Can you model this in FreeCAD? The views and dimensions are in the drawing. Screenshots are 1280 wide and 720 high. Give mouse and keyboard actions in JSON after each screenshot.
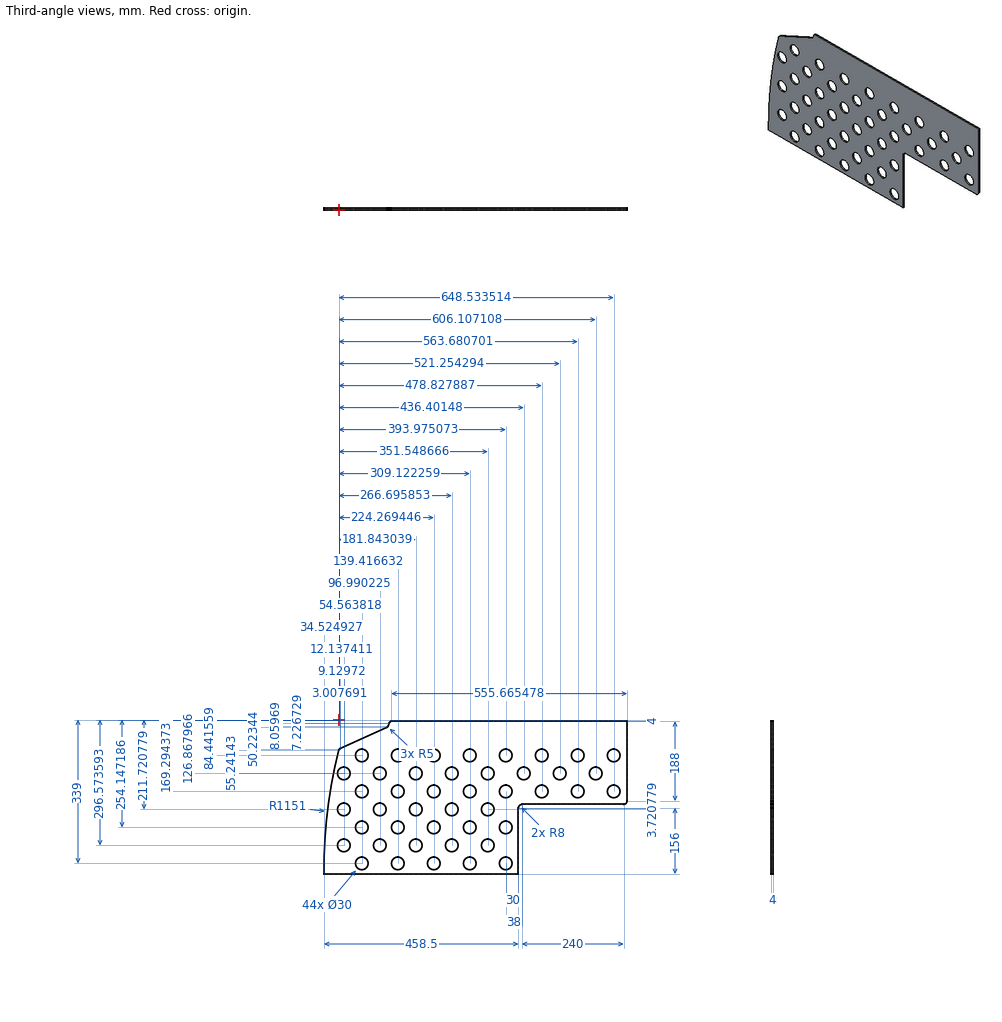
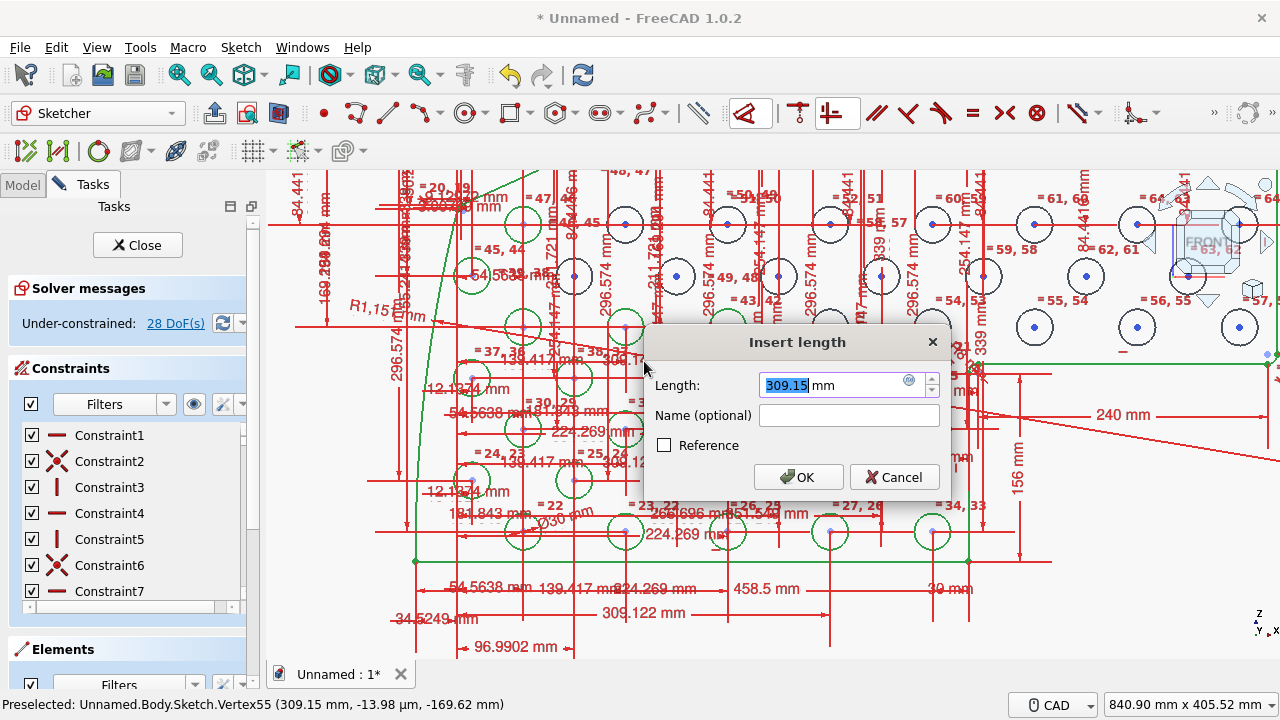
{"action": "type", "text": "309.122259"}
{"action": "key", "text": "Return"}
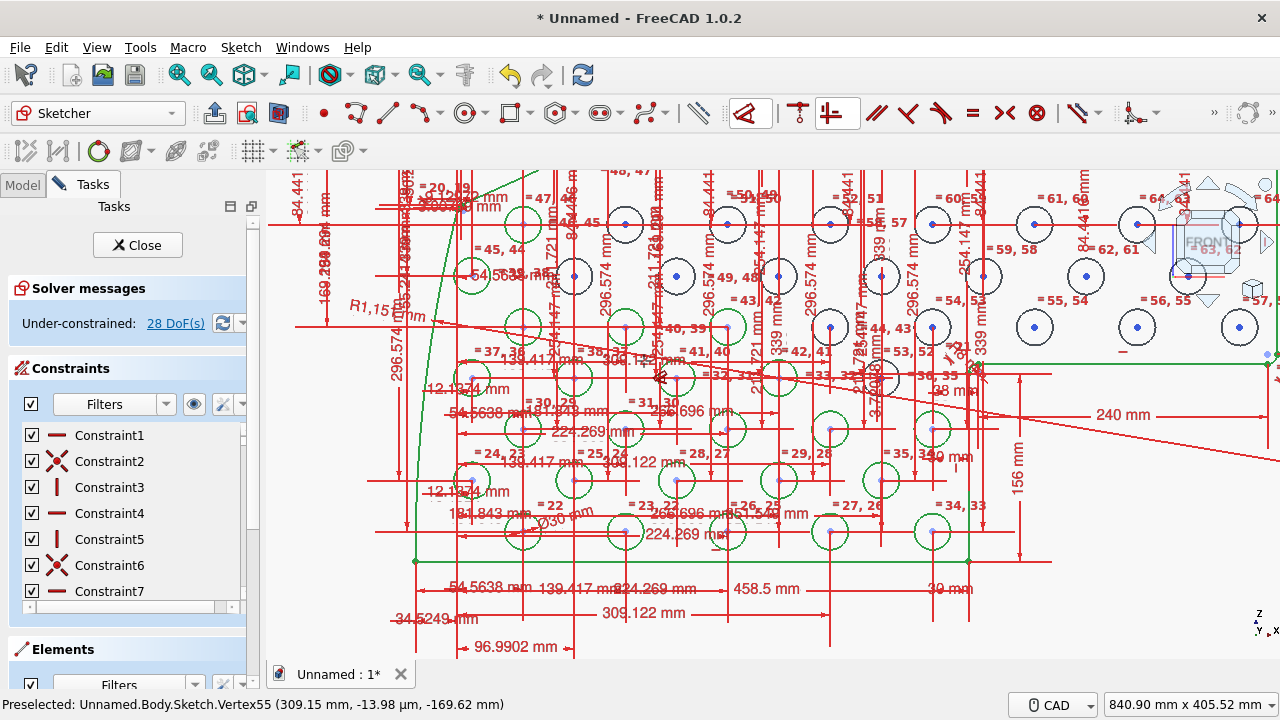
{"action": "left_click", "coordinate": [830, 327]}
{"action": "left_click", "coordinate": [303, 292]}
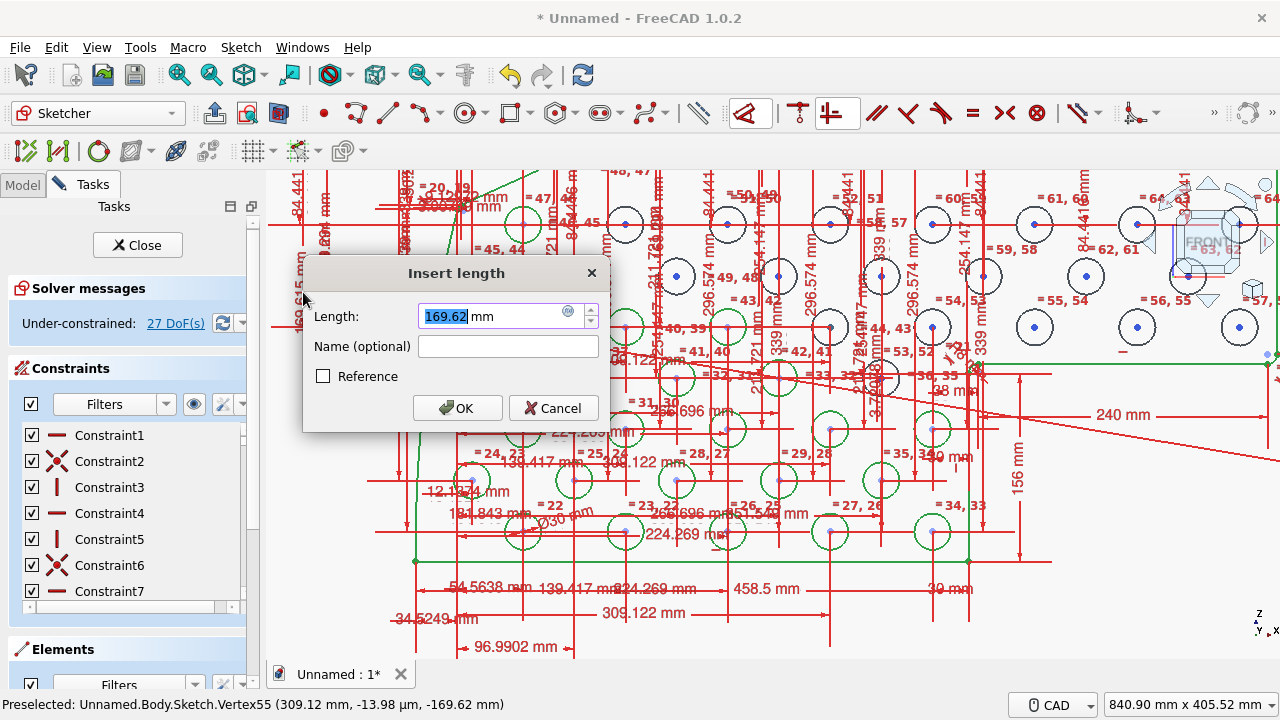
{"action": "type", "text": "169.294373"}
{"action": "key", "text": "Return"}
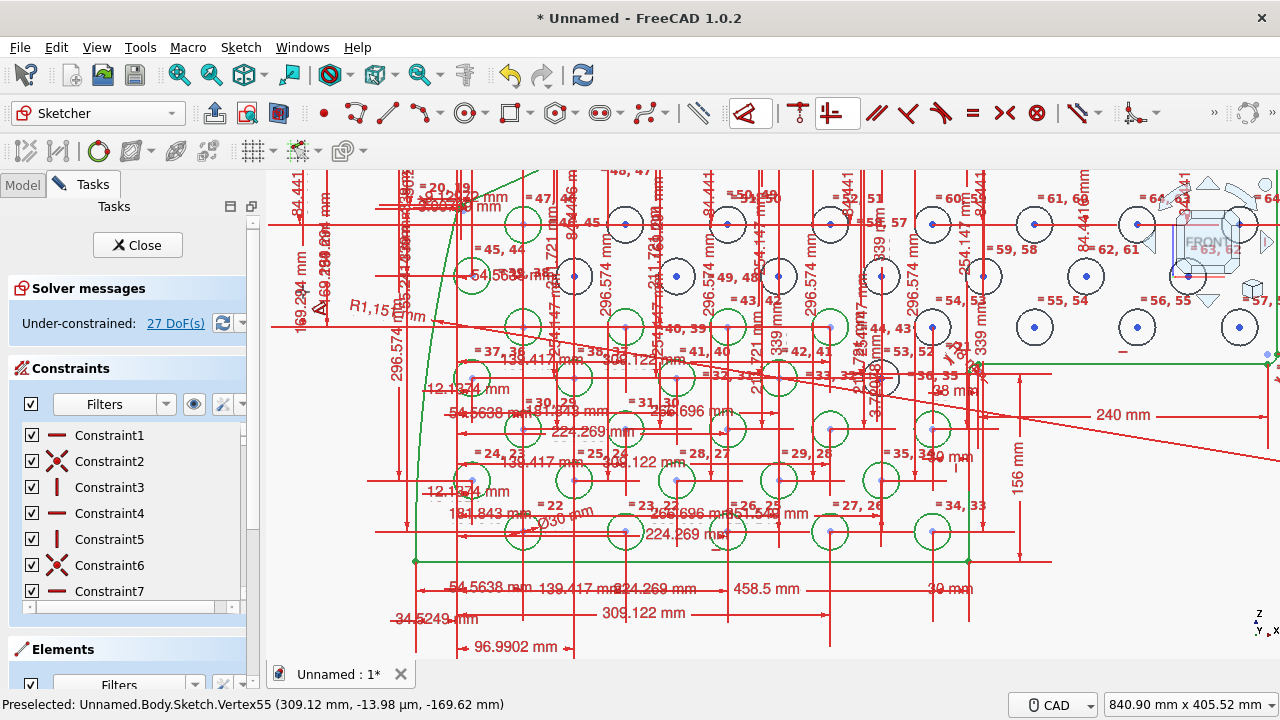
{"action": "left_click", "coordinate": [574, 277]}
{"action": "left_click", "coordinate": [375, 210]}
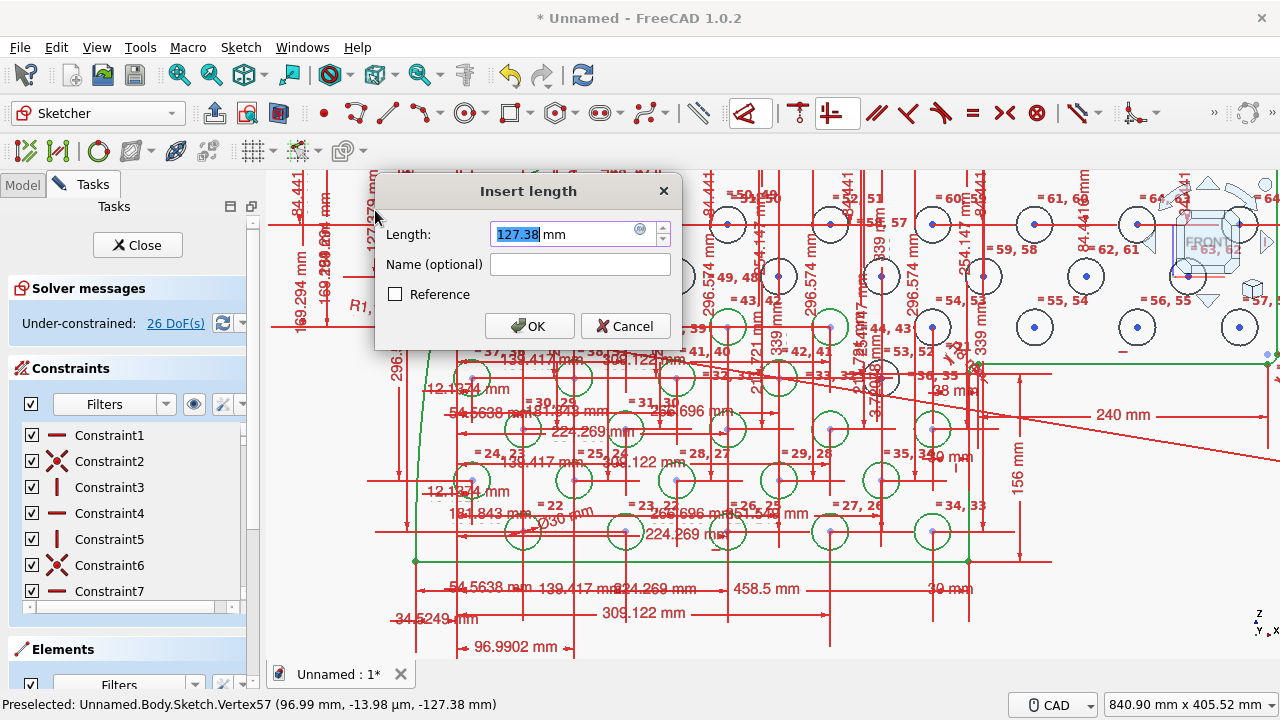
{"action": "type", "text": "126.867966"}
{"action": "key", "text": "Return"}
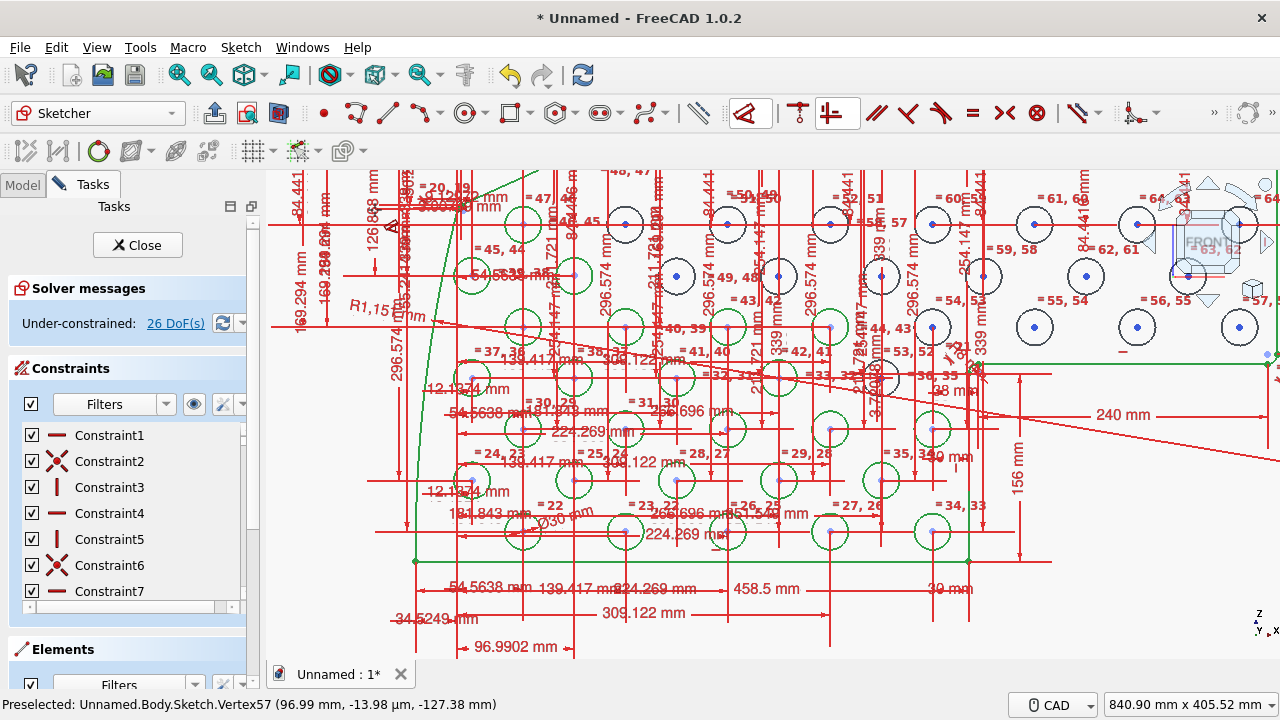
{"action": "left_click", "coordinate": [625, 225]}
{"action": "left_click", "coordinate": [483, 307]}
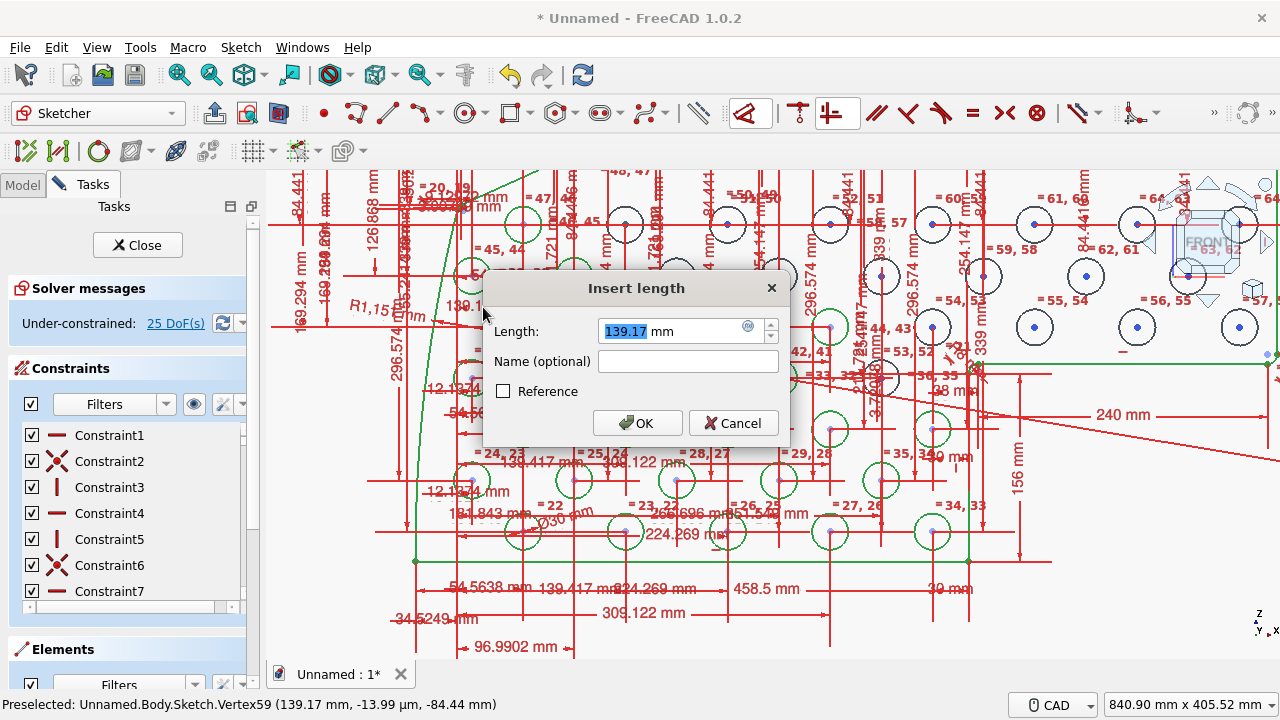
{"action": "type", "text": "139.416632"}
{"action": "key", "text": "Return"}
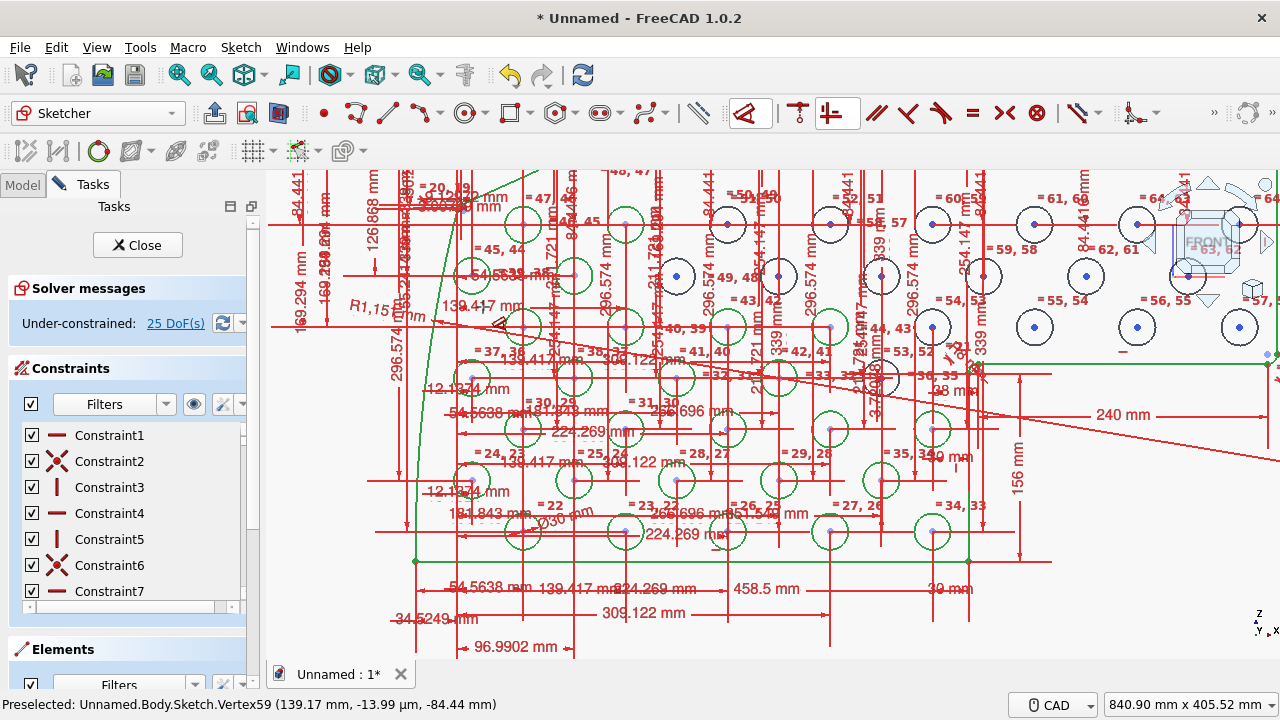
{"action": "left_click", "coordinate": [677, 277]}
{"action": "left_click", "coordinate": [567, 335]}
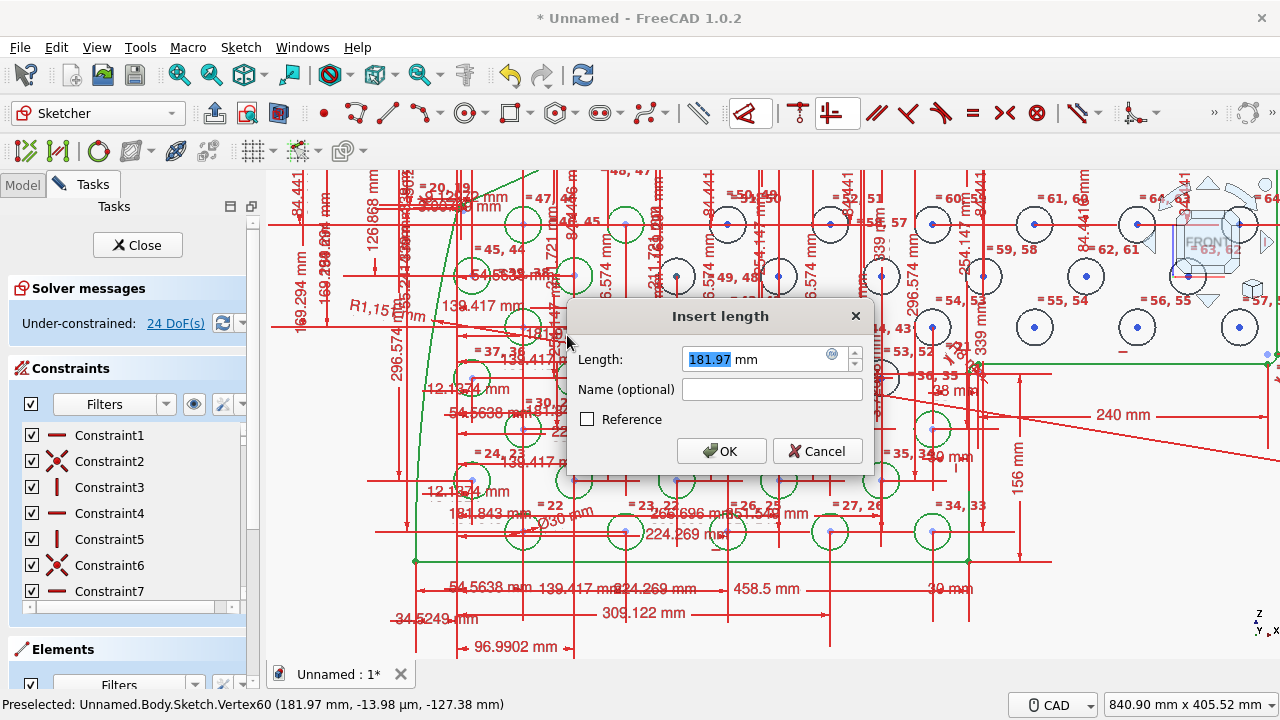
{"action": "type", "text": "181.843039"}
{"action": "key", "text": "Return"}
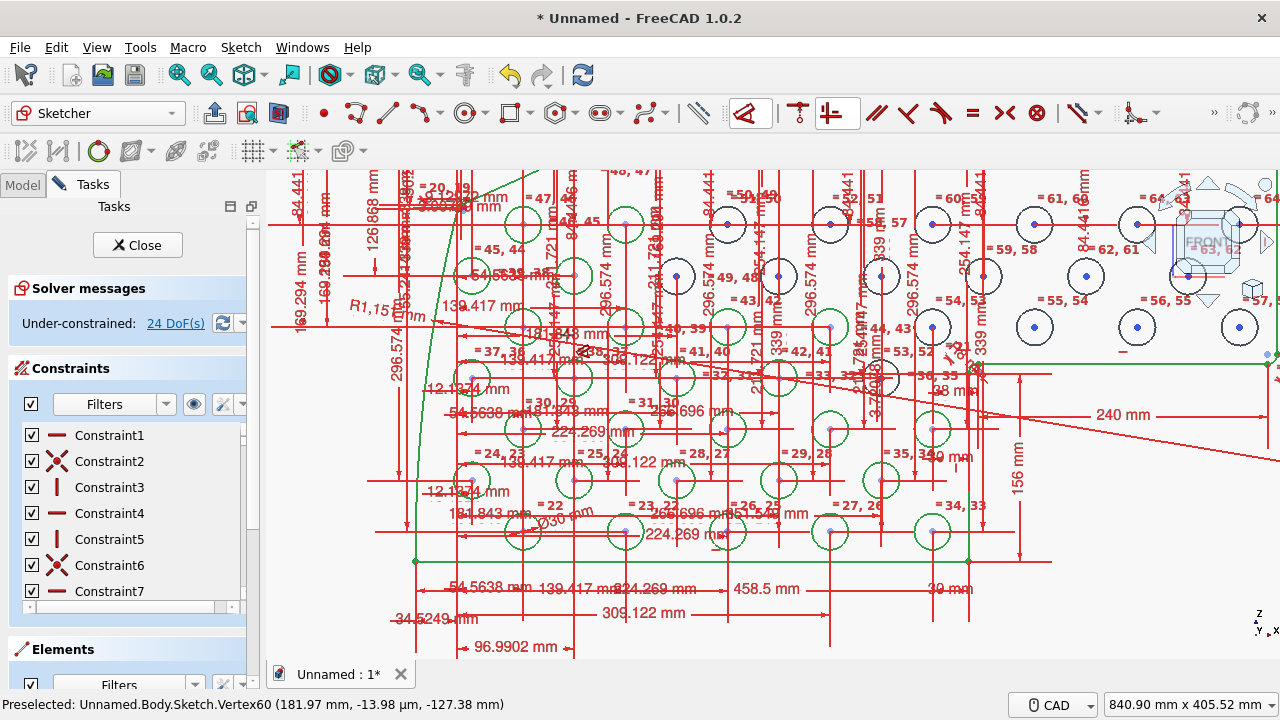
{"action": "left_click", "coordinate": [677, 277]}
{"action": "left_click", "coordinate": [759, 210]}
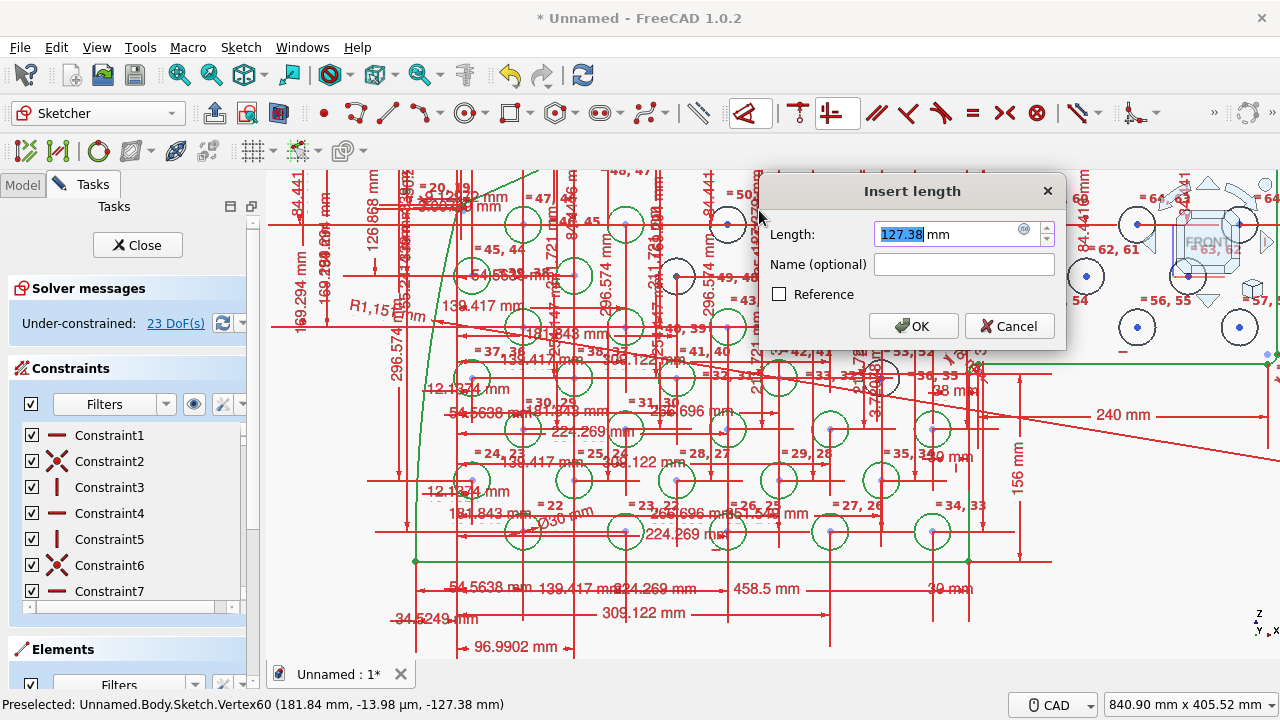
{"action": "type", "text": "126.867966"}
{"action": "key", "text": "Return"}